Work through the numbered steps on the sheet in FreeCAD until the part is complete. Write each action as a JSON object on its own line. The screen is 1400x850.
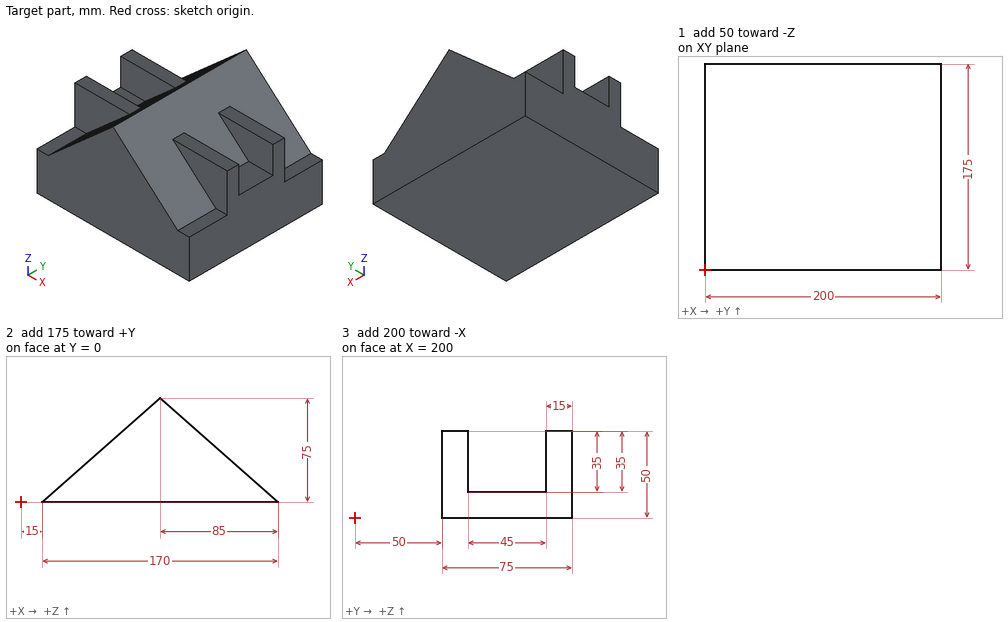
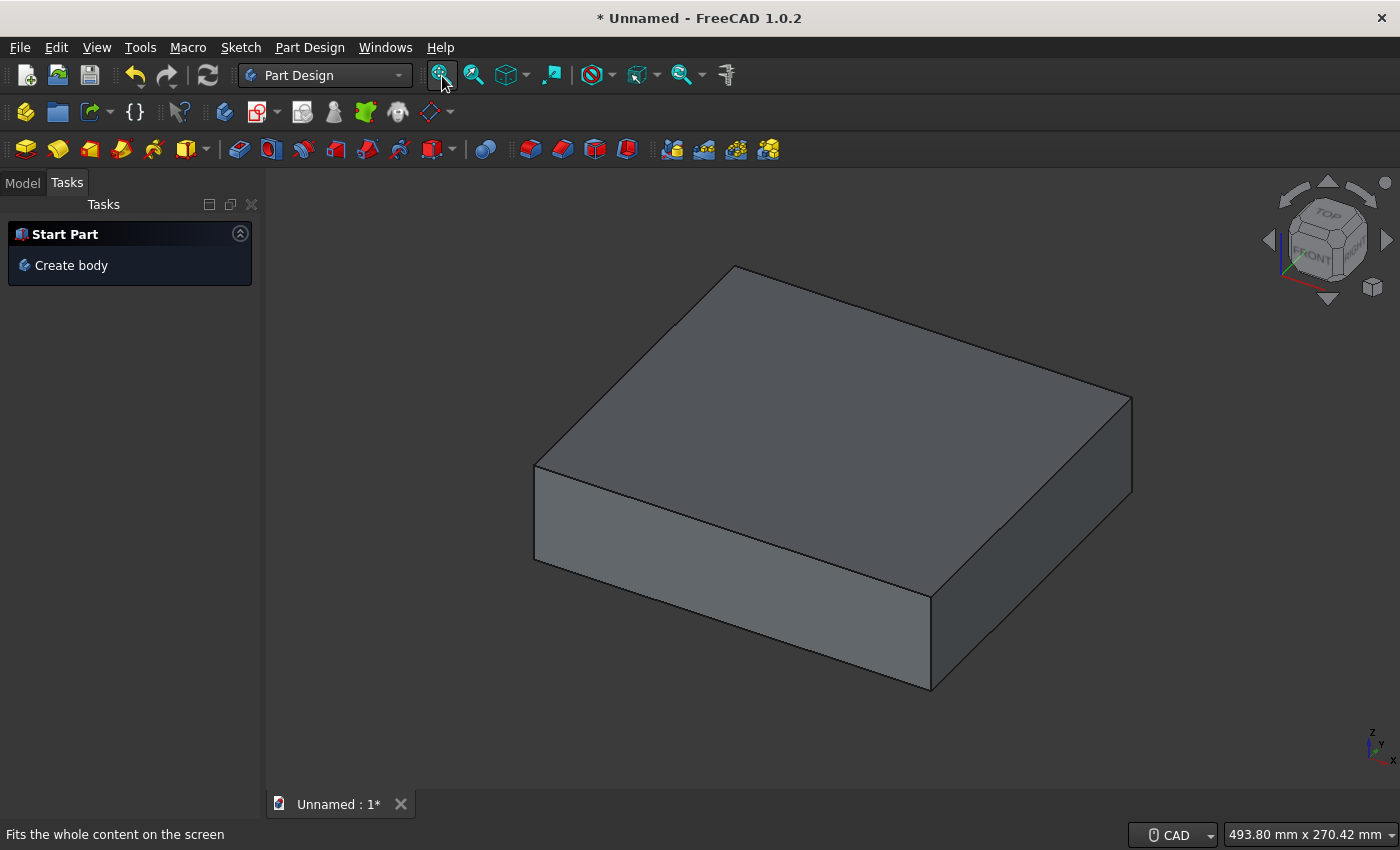
{"action": "left_click", "coordinate": [846, 615]}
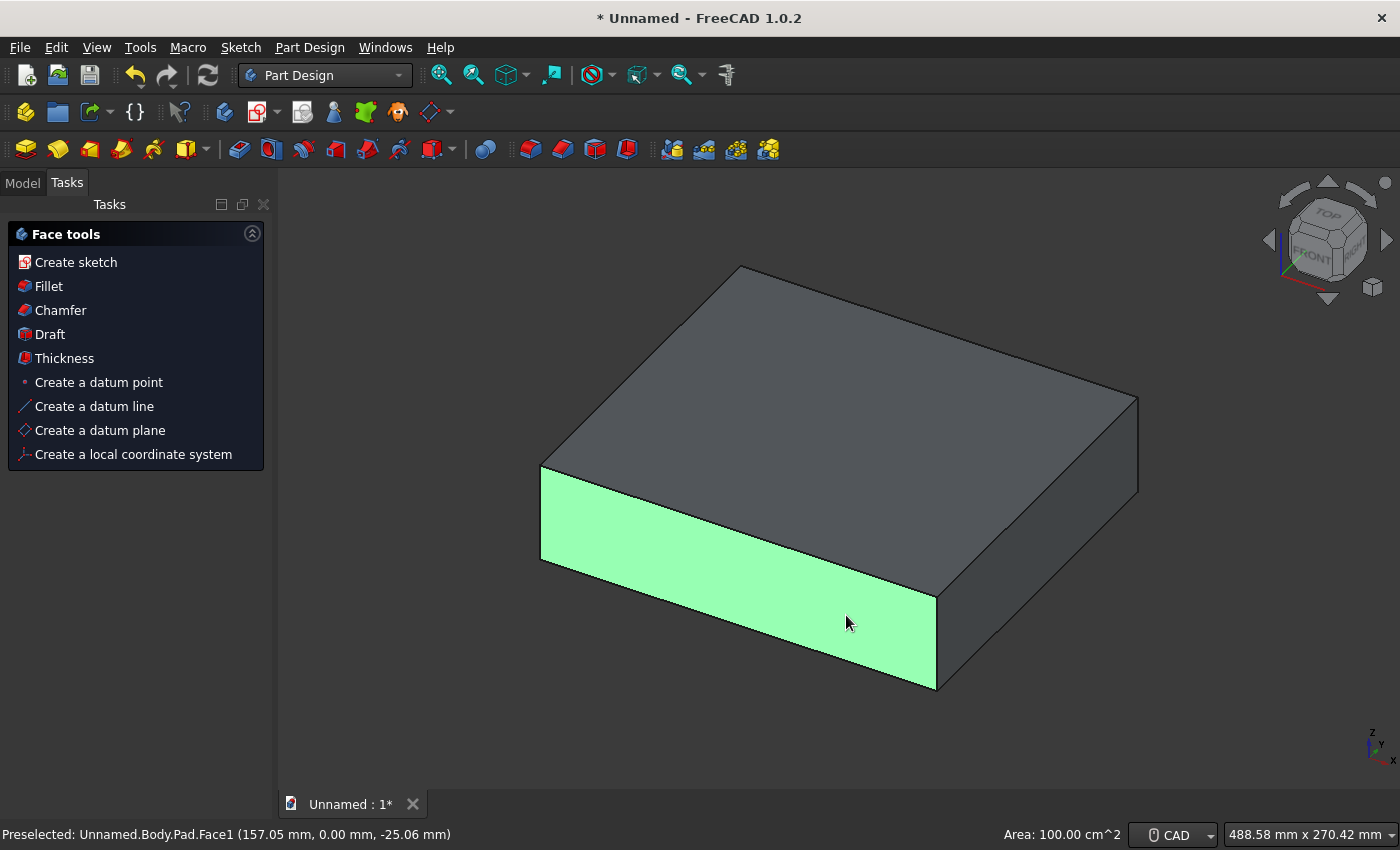
{"action": "left_click", "coordinate": [258, 112]}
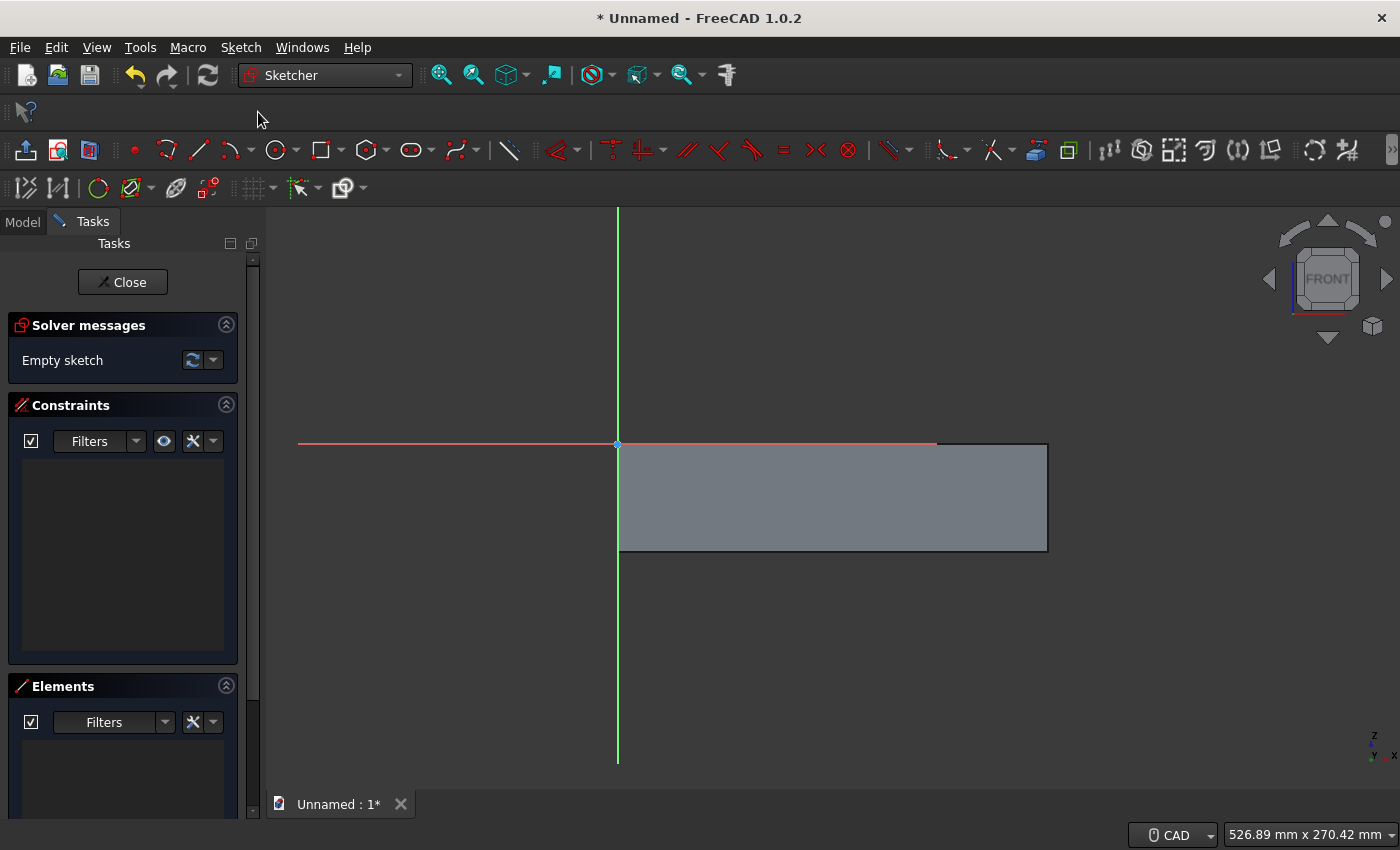
{"action": "scroll", "coordinate": [881, 235], "scroll_direction": "up", "scroll_amount": 3}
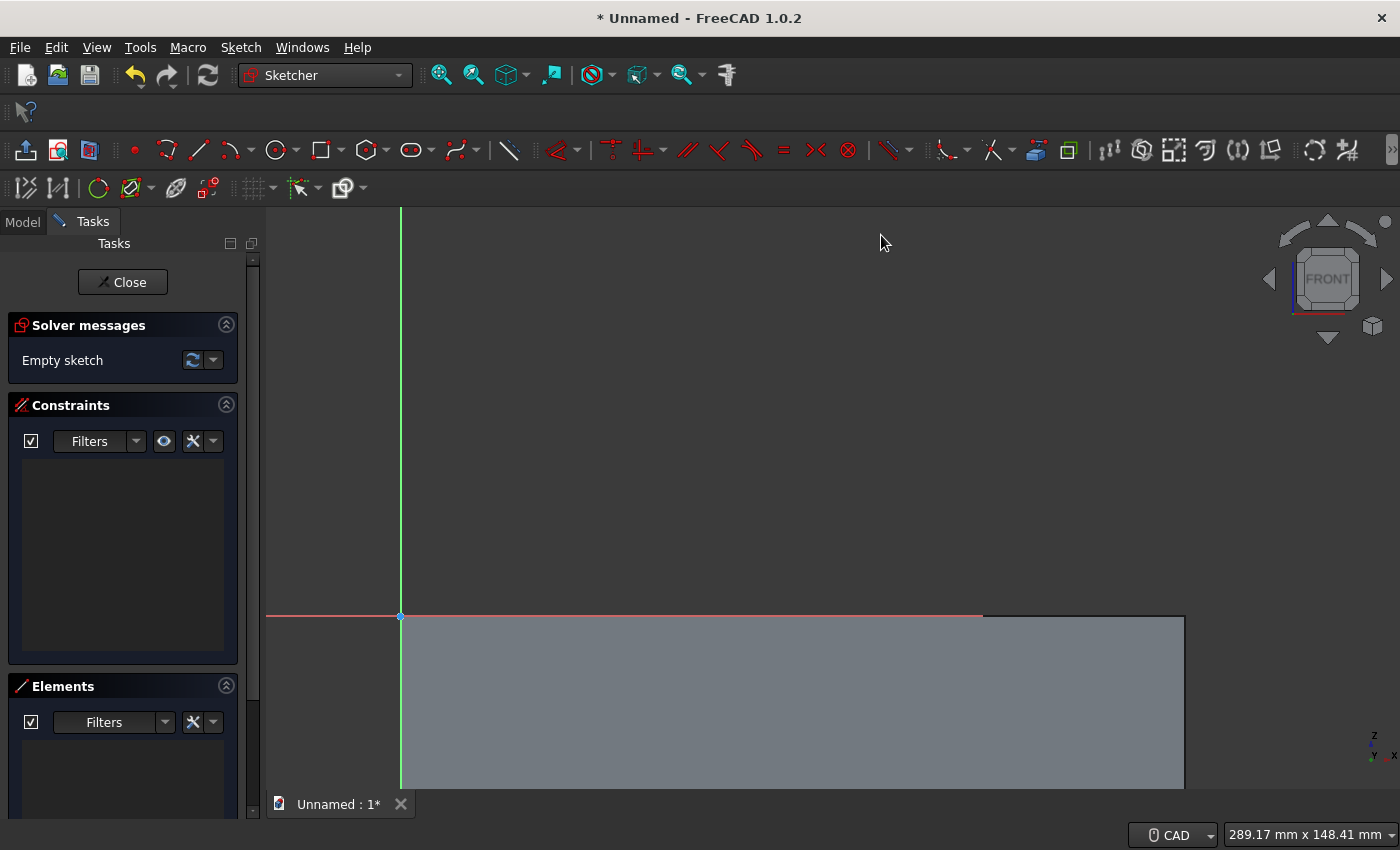
{"action": "left_click", "coordinate": [168, 150]}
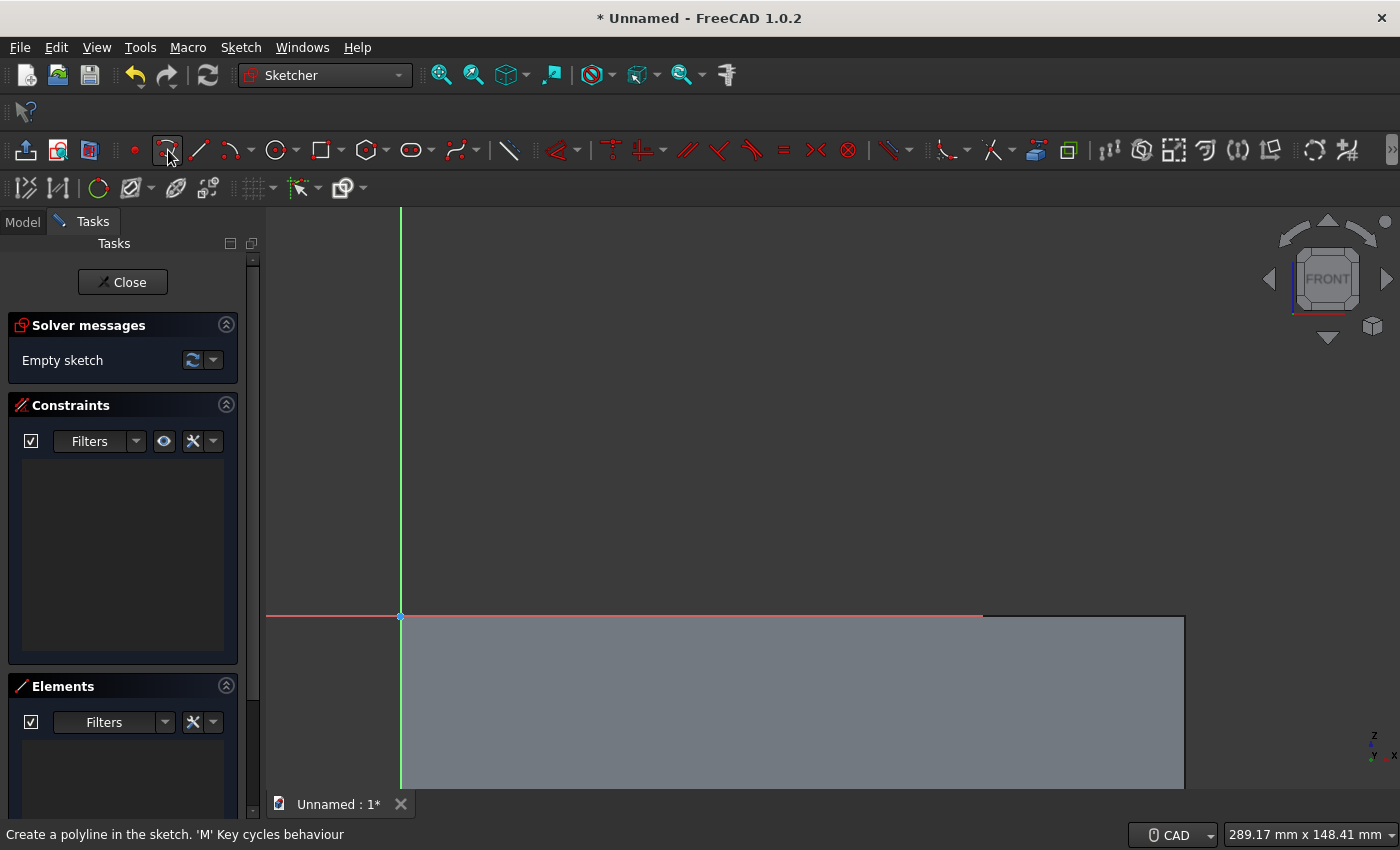
{"action": "left_click", "coordinate": [460, 616]}
{"action": "left_click", "coordinate": [1126, 607]}
{"action": "left_click", "coordinate": [793, 322]}
{"action": "left_click", "coordinate": [460, 616]}
{"action": "key", "text": "Escape"}
{"action": "key", "text": "Escape"}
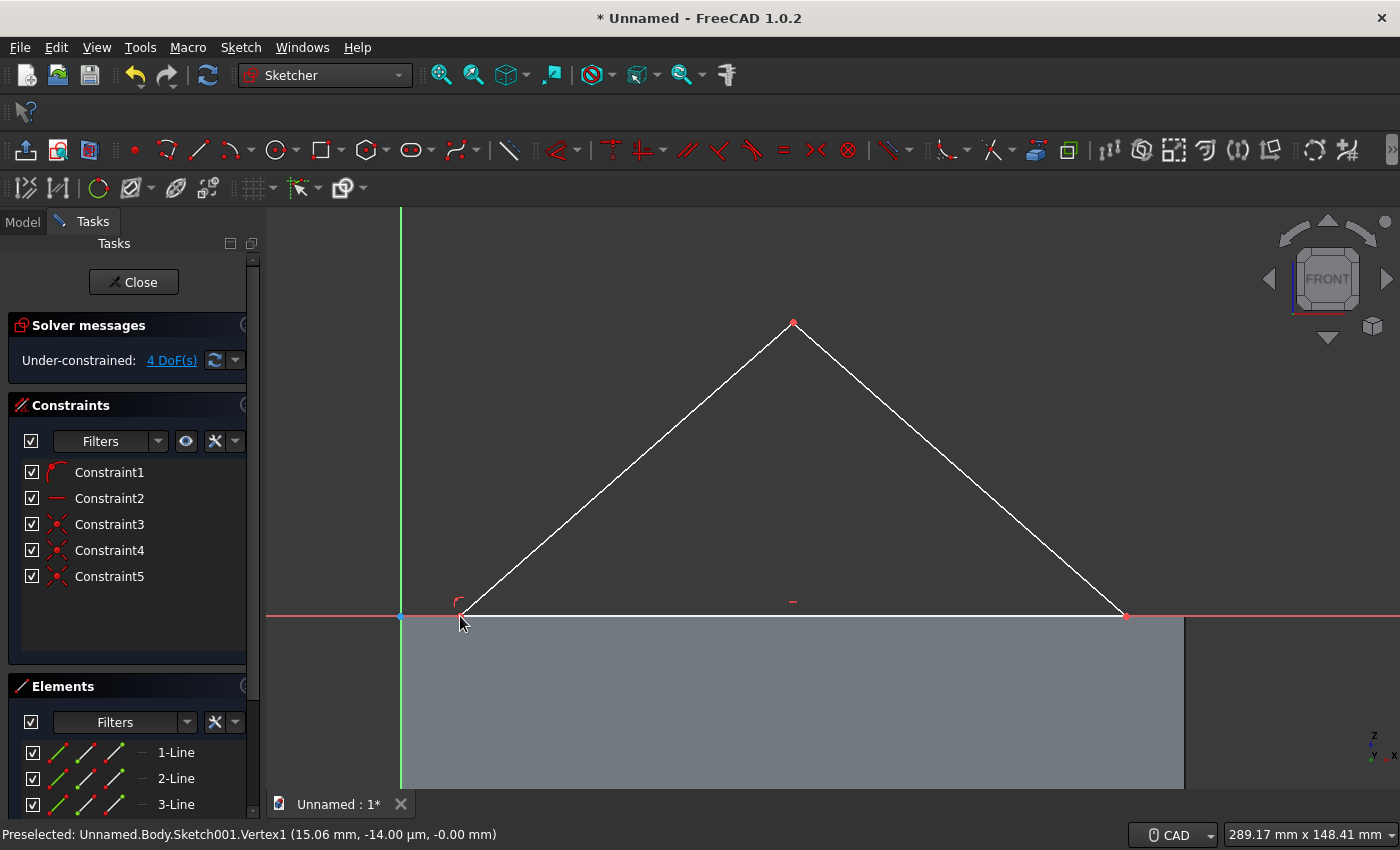
{"action": "left_click", "coordinate": [556, 150]}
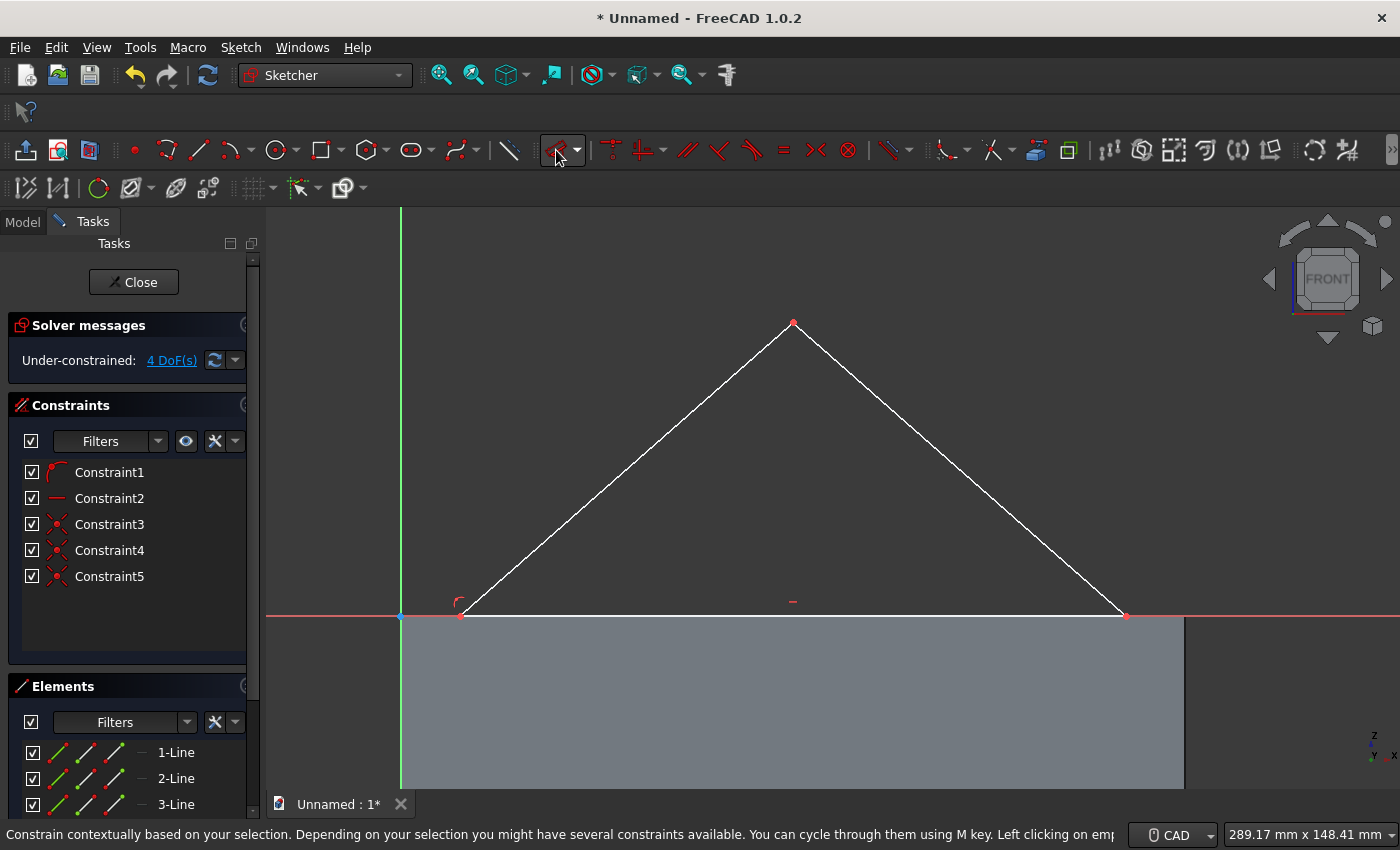
{"action": "left_click", "coordinate": [660, 616]}
{"action": "left_click", "coordinate": [793, 650]}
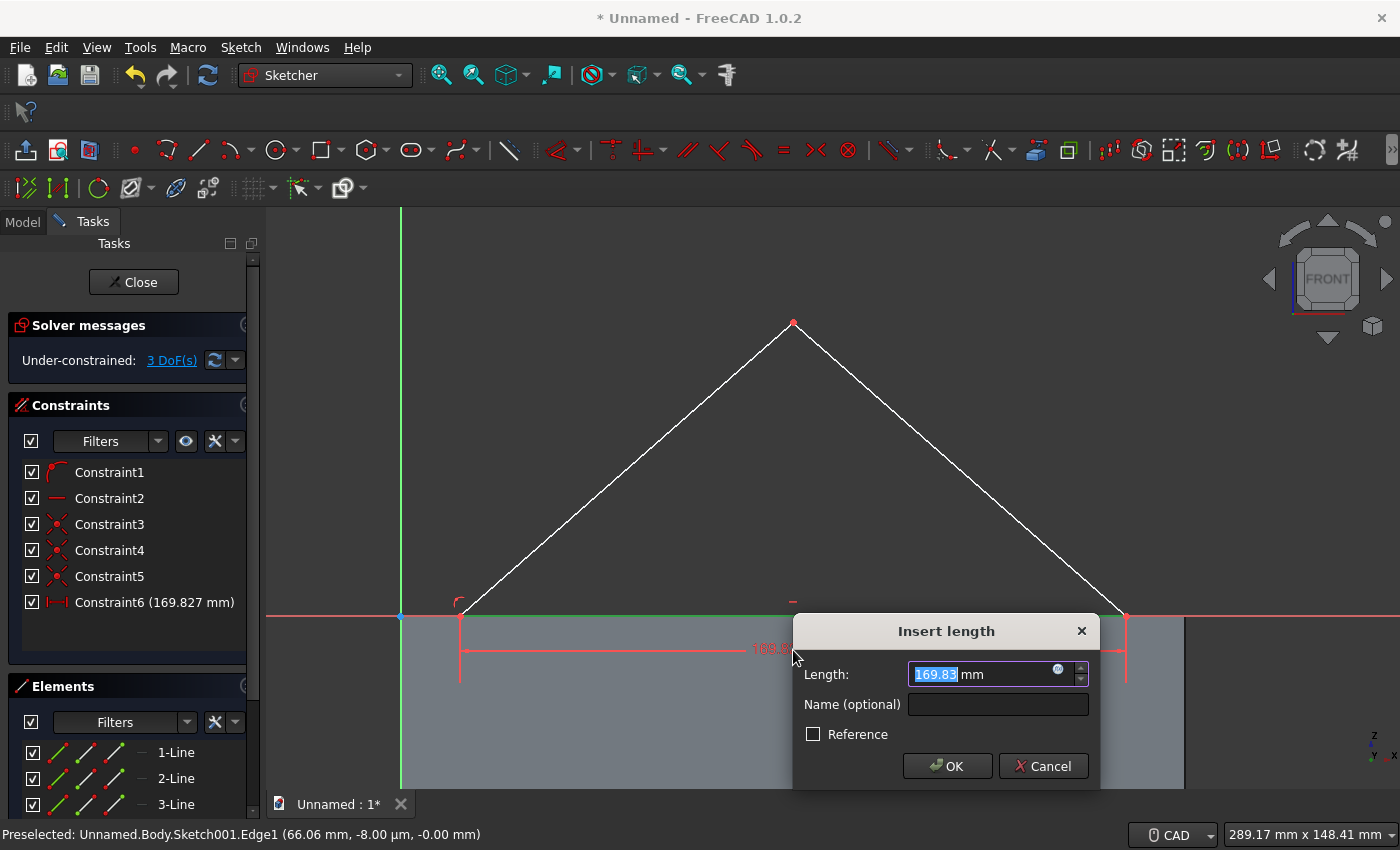
{"action": "type", "text": "170"}
{"action": "key", "text": "Return"}